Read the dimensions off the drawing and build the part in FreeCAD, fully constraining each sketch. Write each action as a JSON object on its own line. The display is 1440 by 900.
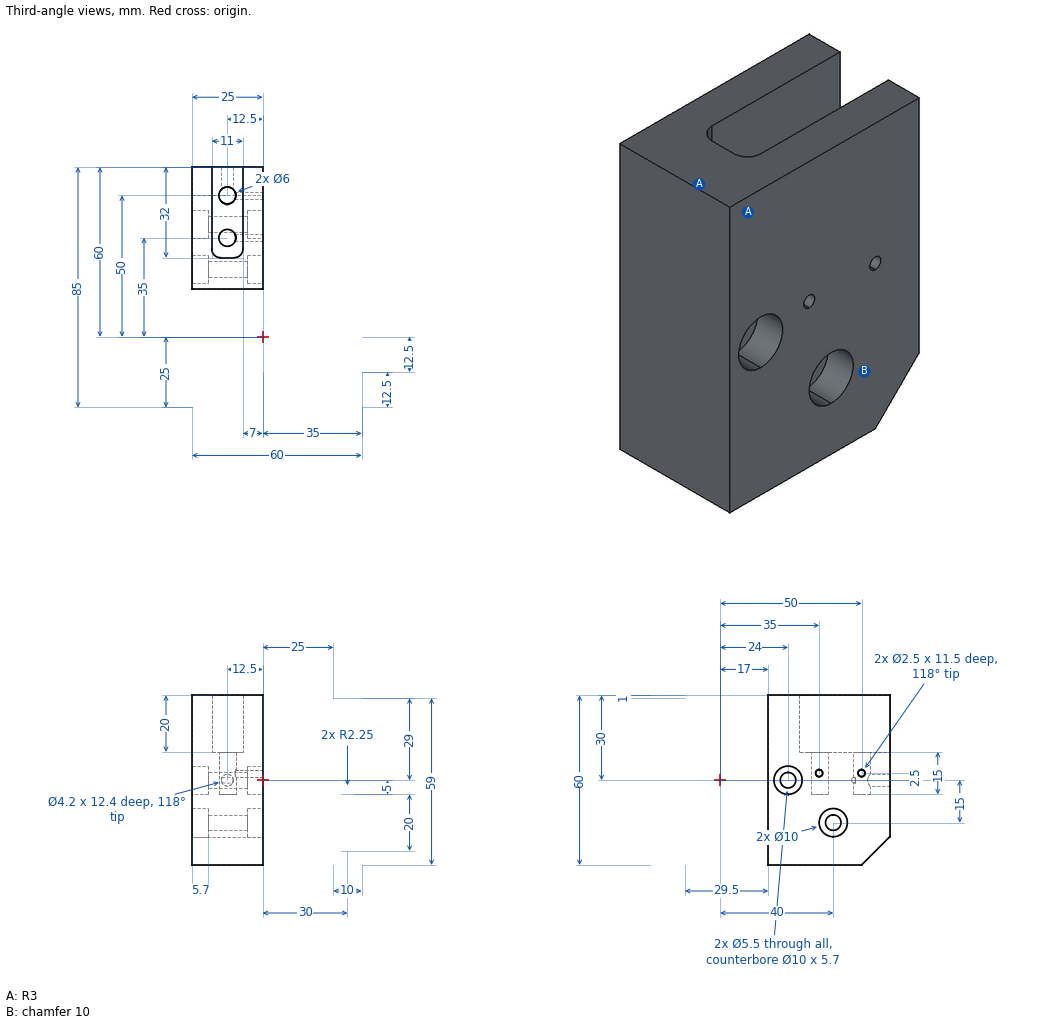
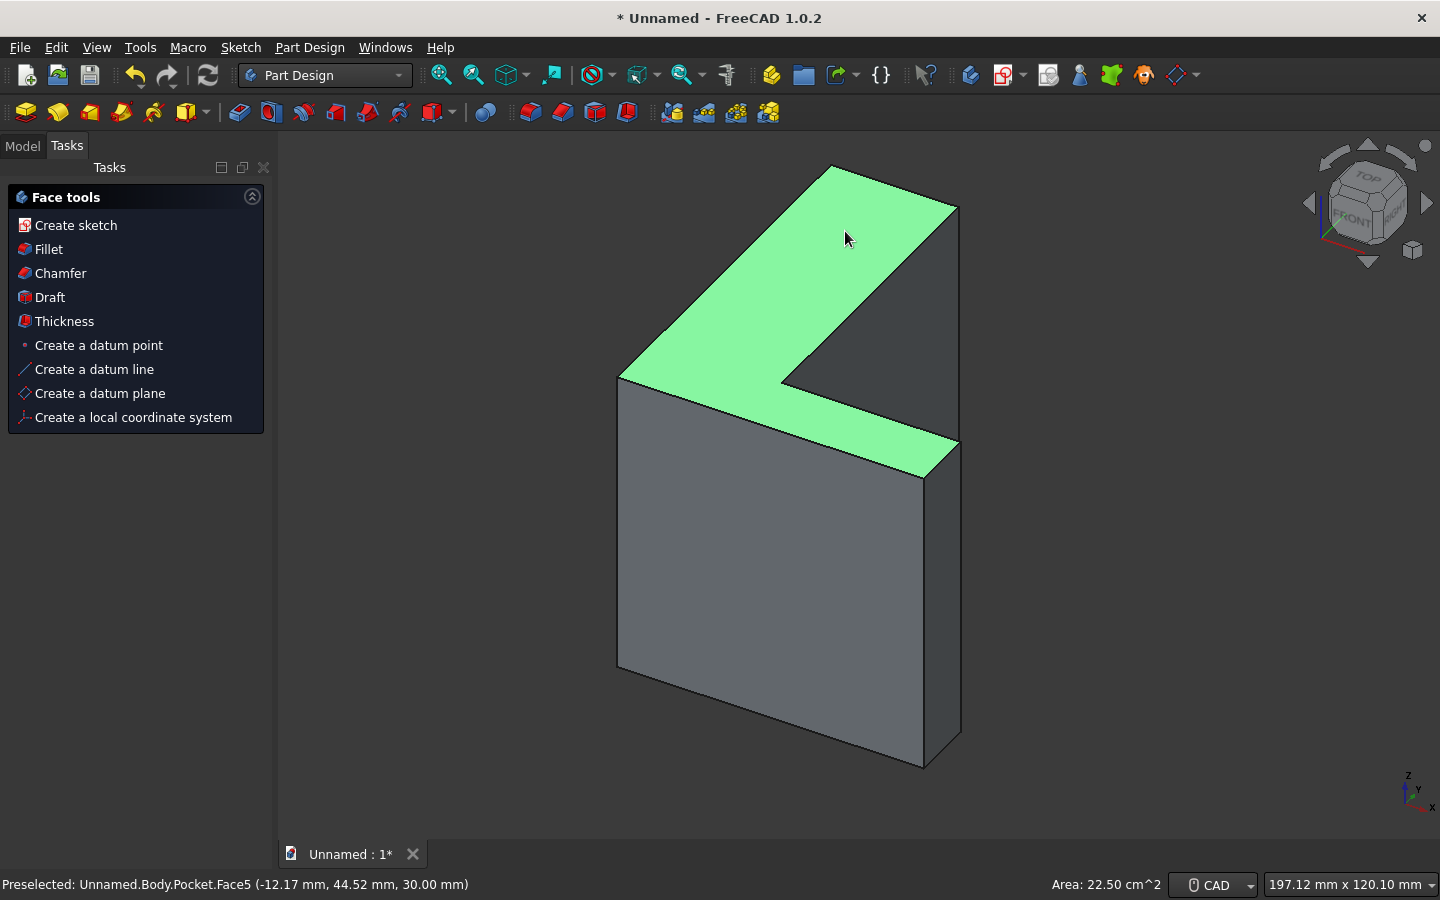
{"action": "left_click", "coordinate": [1004, 76]}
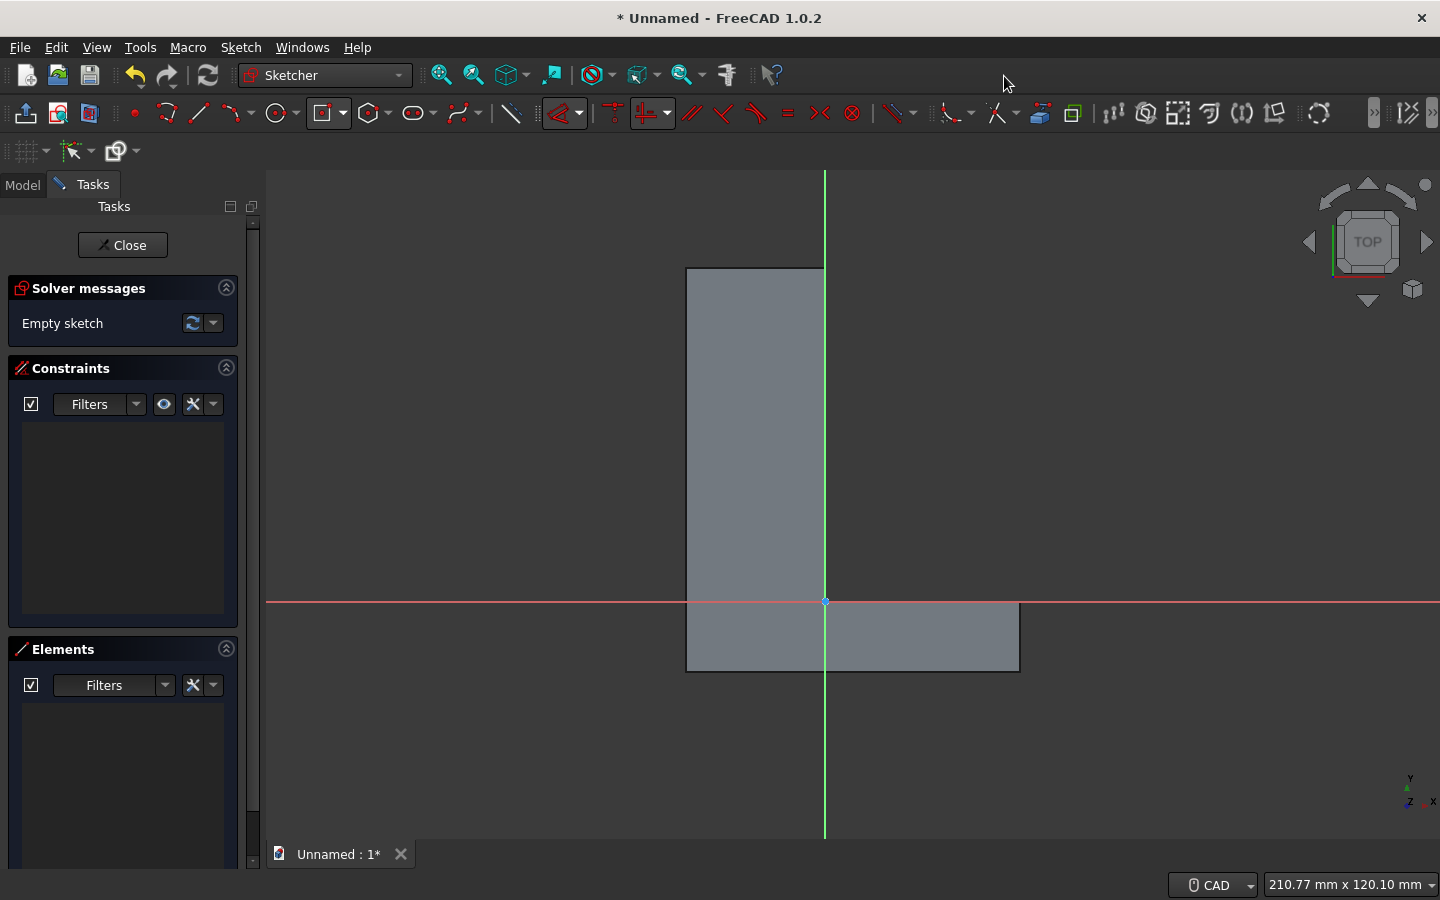
{"action": "left_click", "coordinate": [346, 114]}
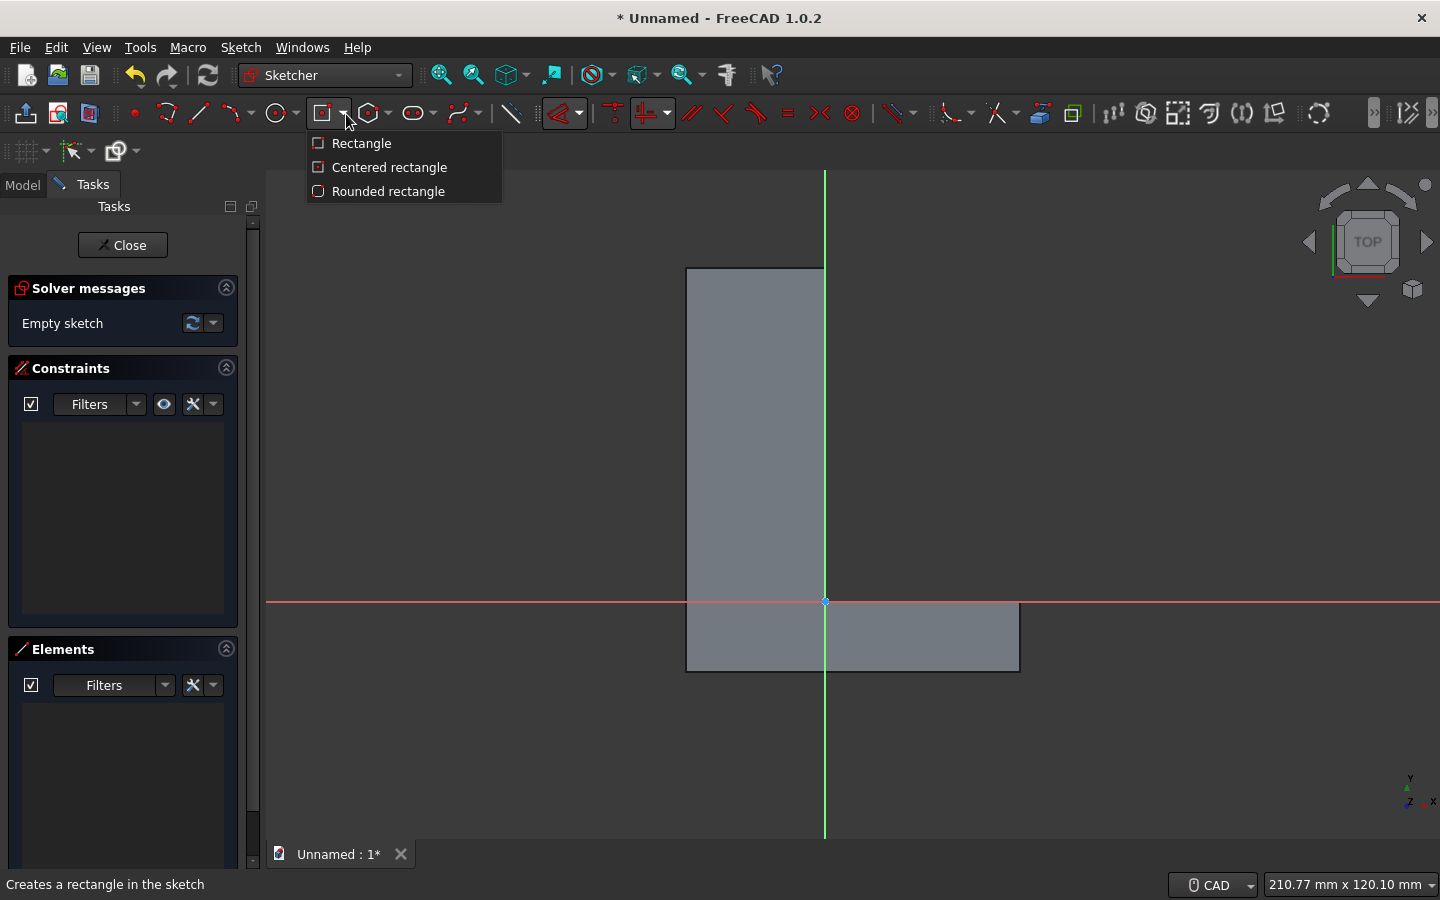
{"action": "left_click", "coordinate": [404, 143]}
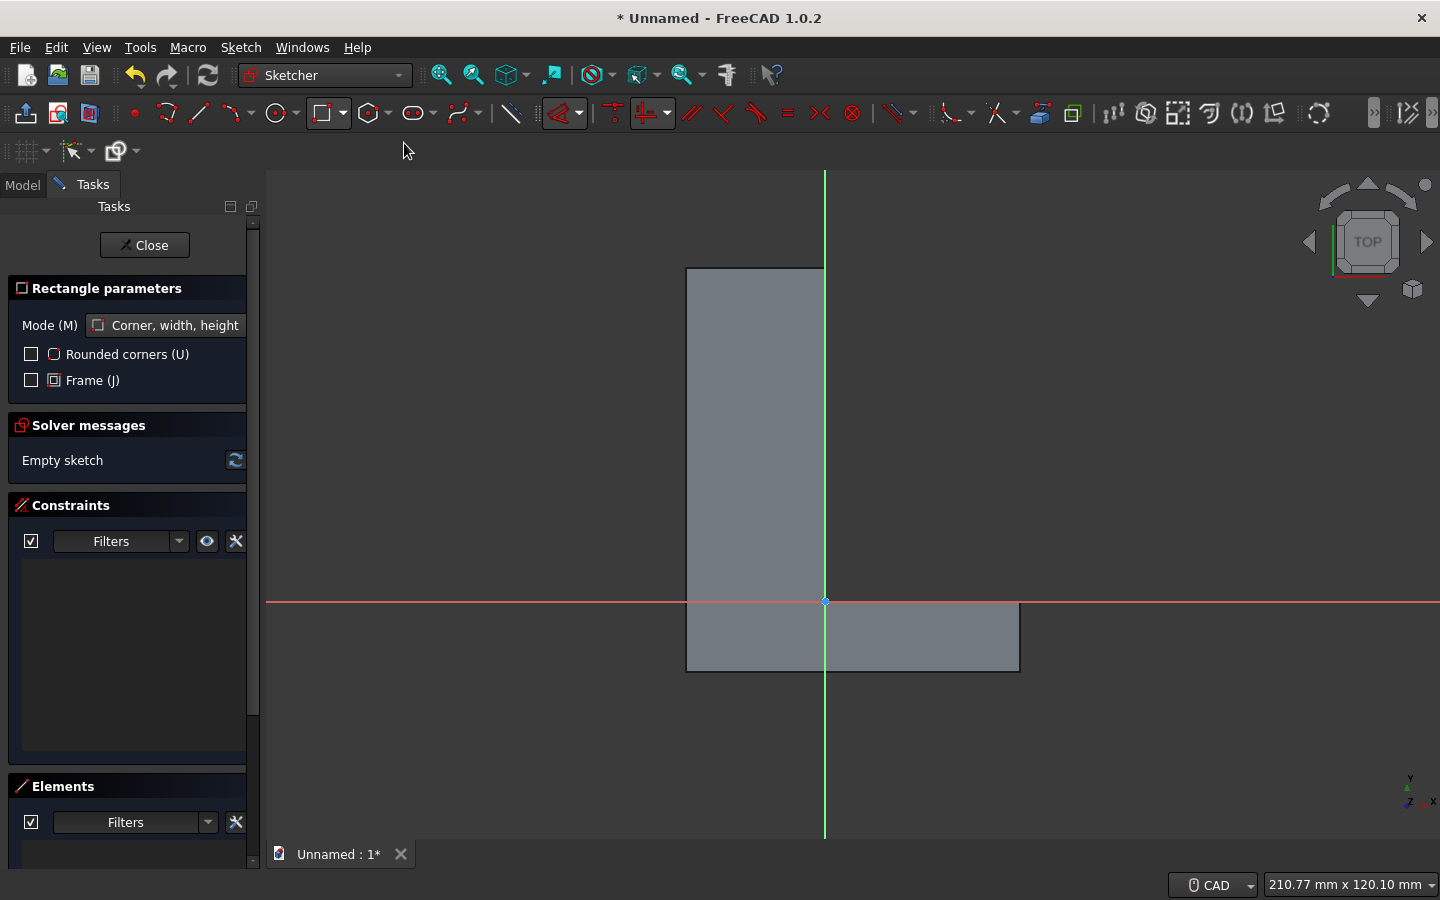
{"action": "left_click", "coordinate": [725, 268]}
{"action": "mouse_move", "coordinate": [786, 446]}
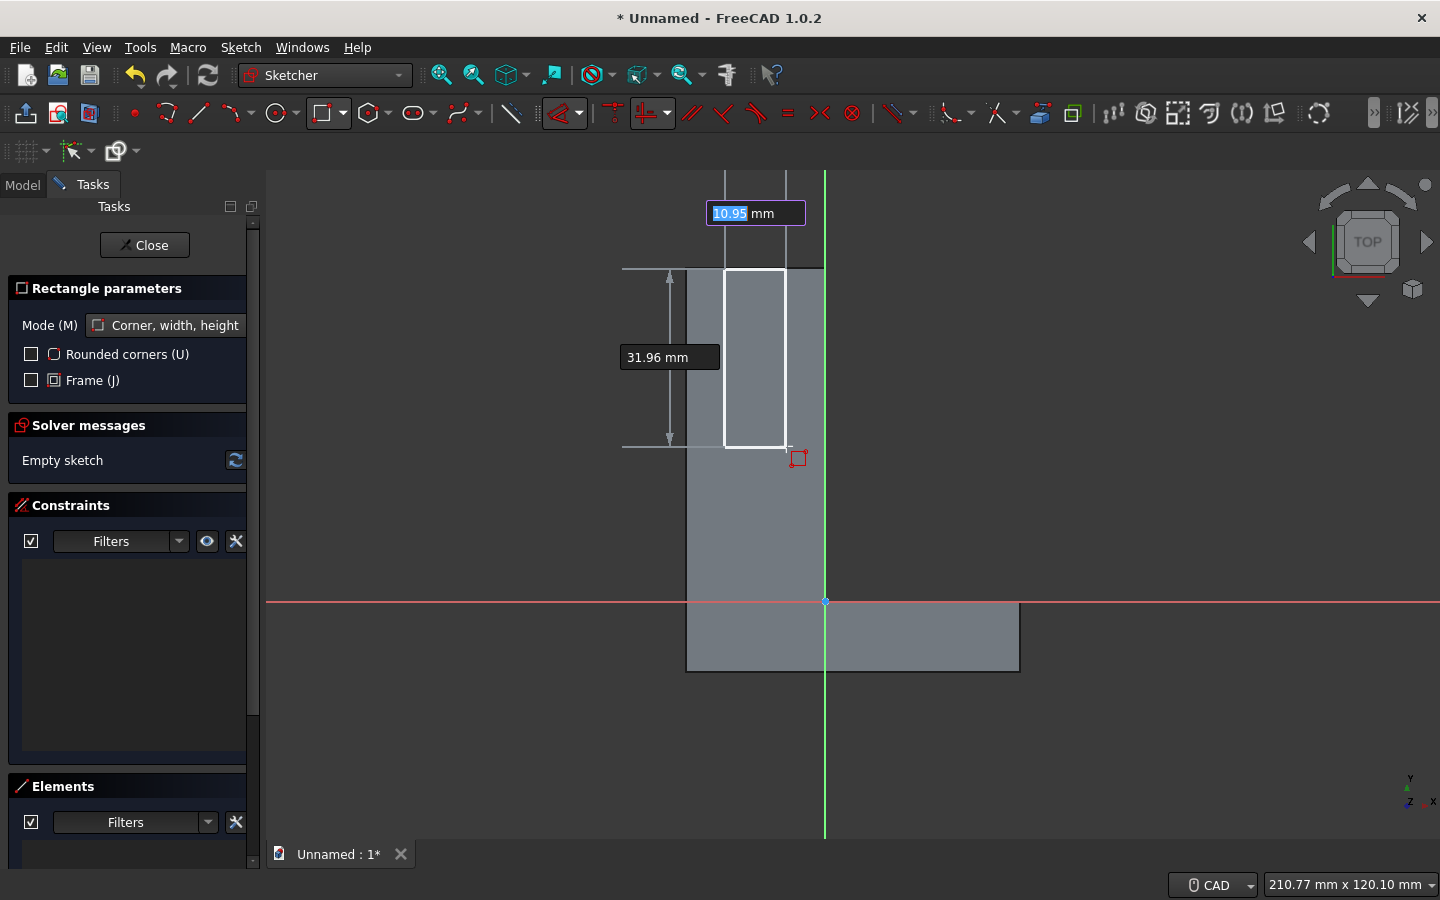
{"action": "type", "text": "11"}
{"action": "key", "text": "Tab"}
{"action": "type", "text": "32"}
{"action": "key", "text": "Return"}
{"action": "key", "text": "Escape"}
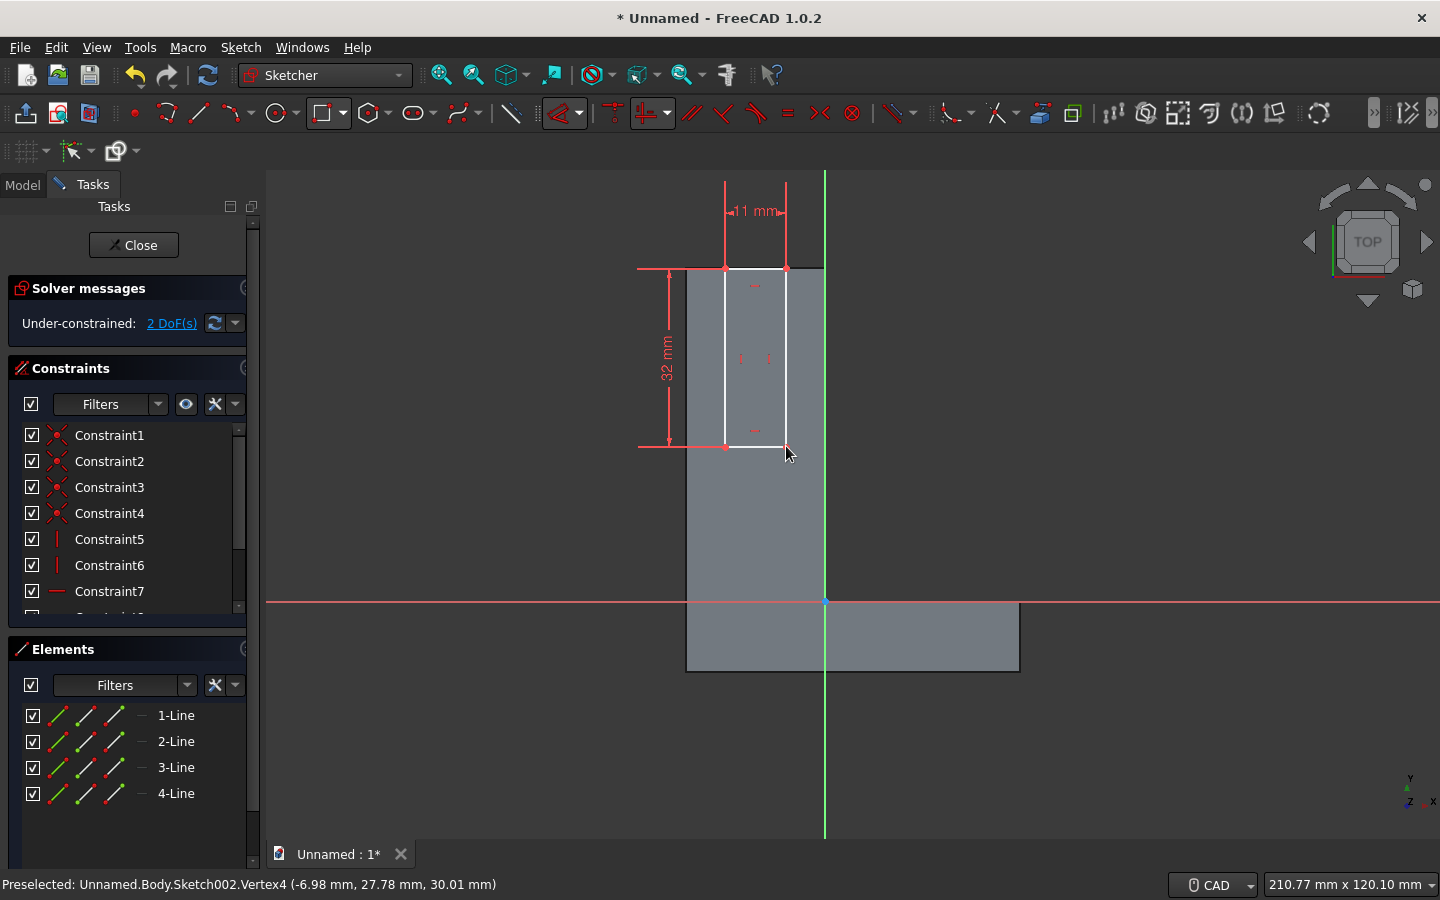
{"action": "left_click", "coordinate": [786, 447]}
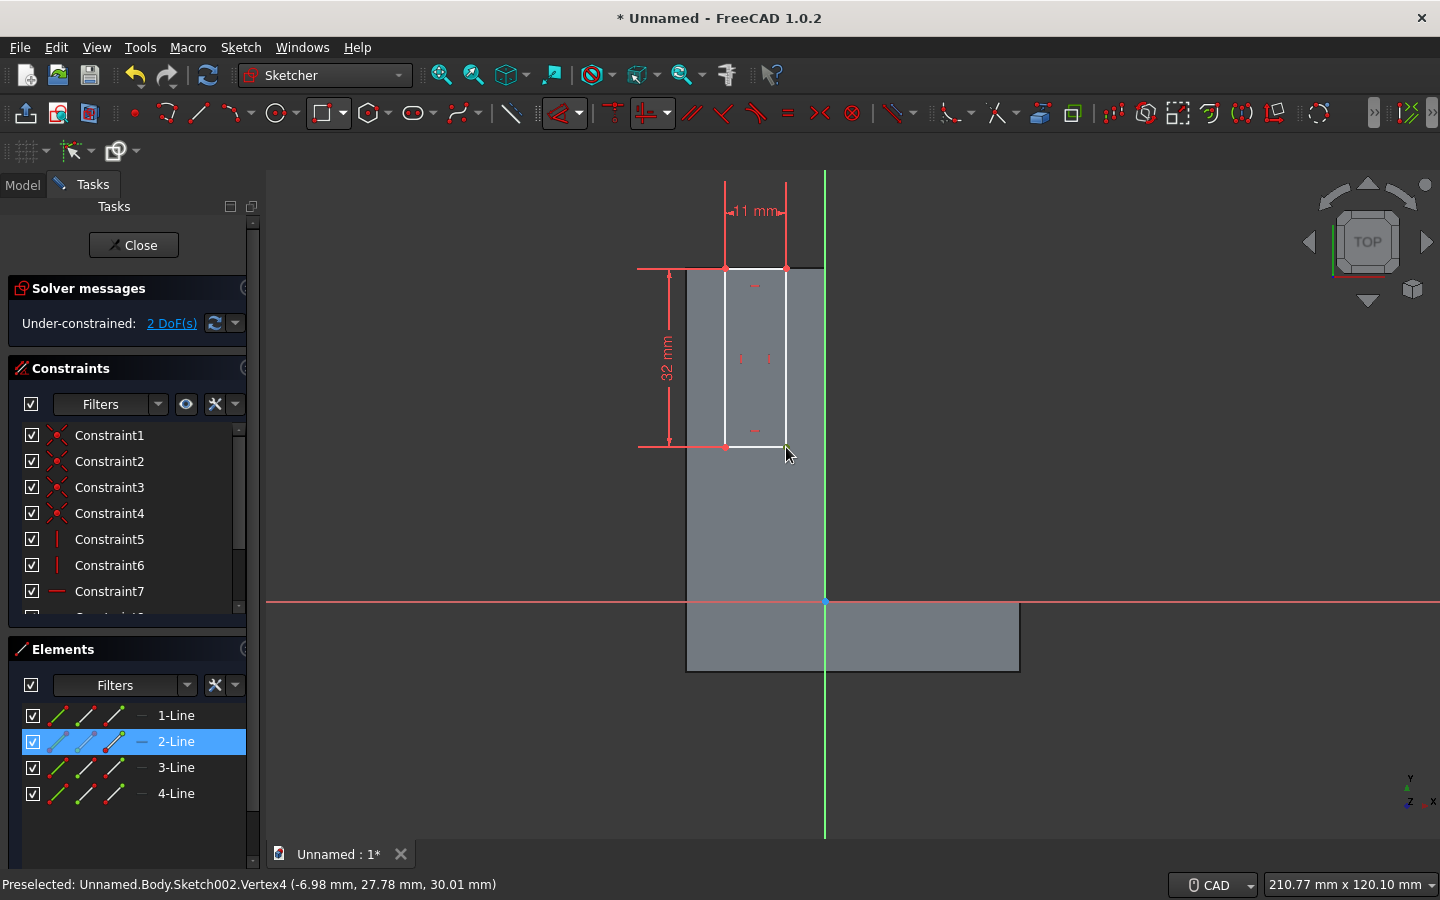
{"action": "left_click", "coordinate": [582, 114]}